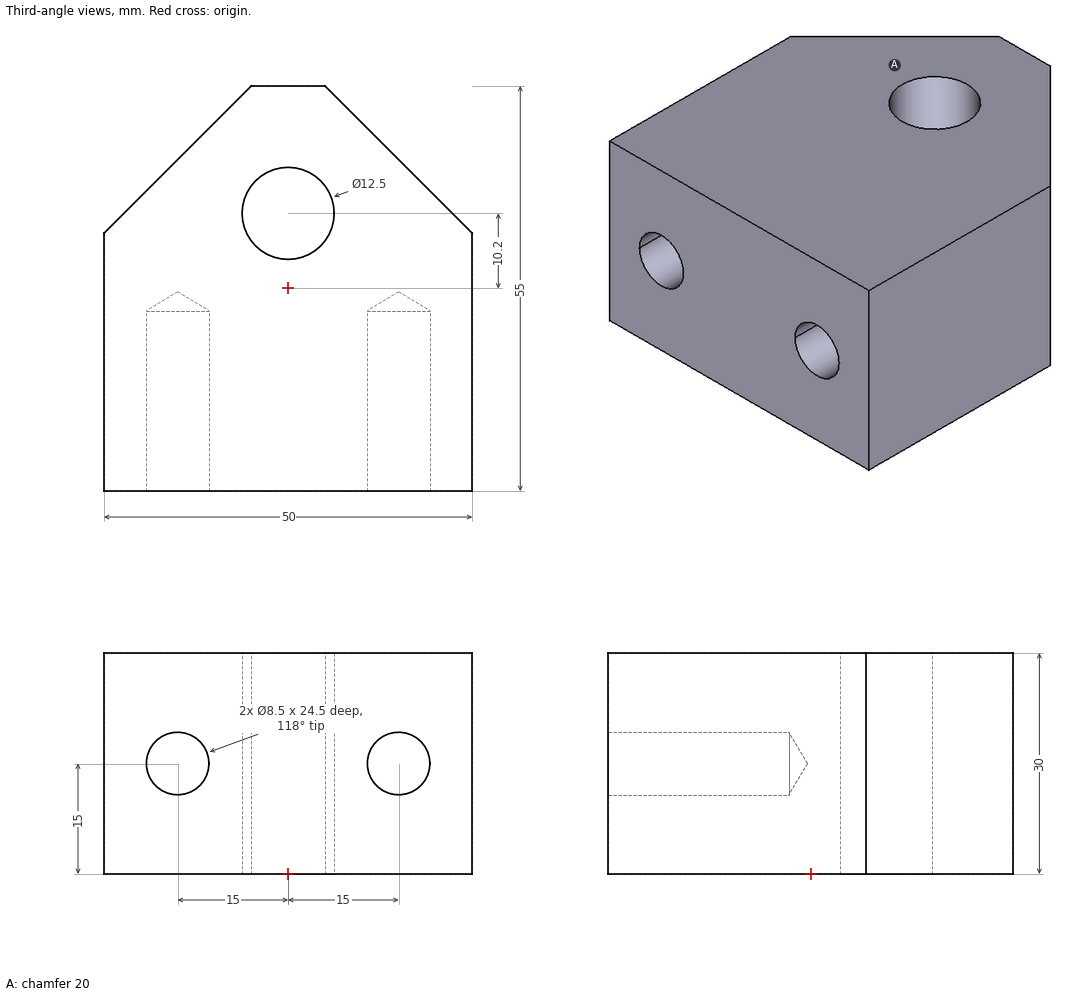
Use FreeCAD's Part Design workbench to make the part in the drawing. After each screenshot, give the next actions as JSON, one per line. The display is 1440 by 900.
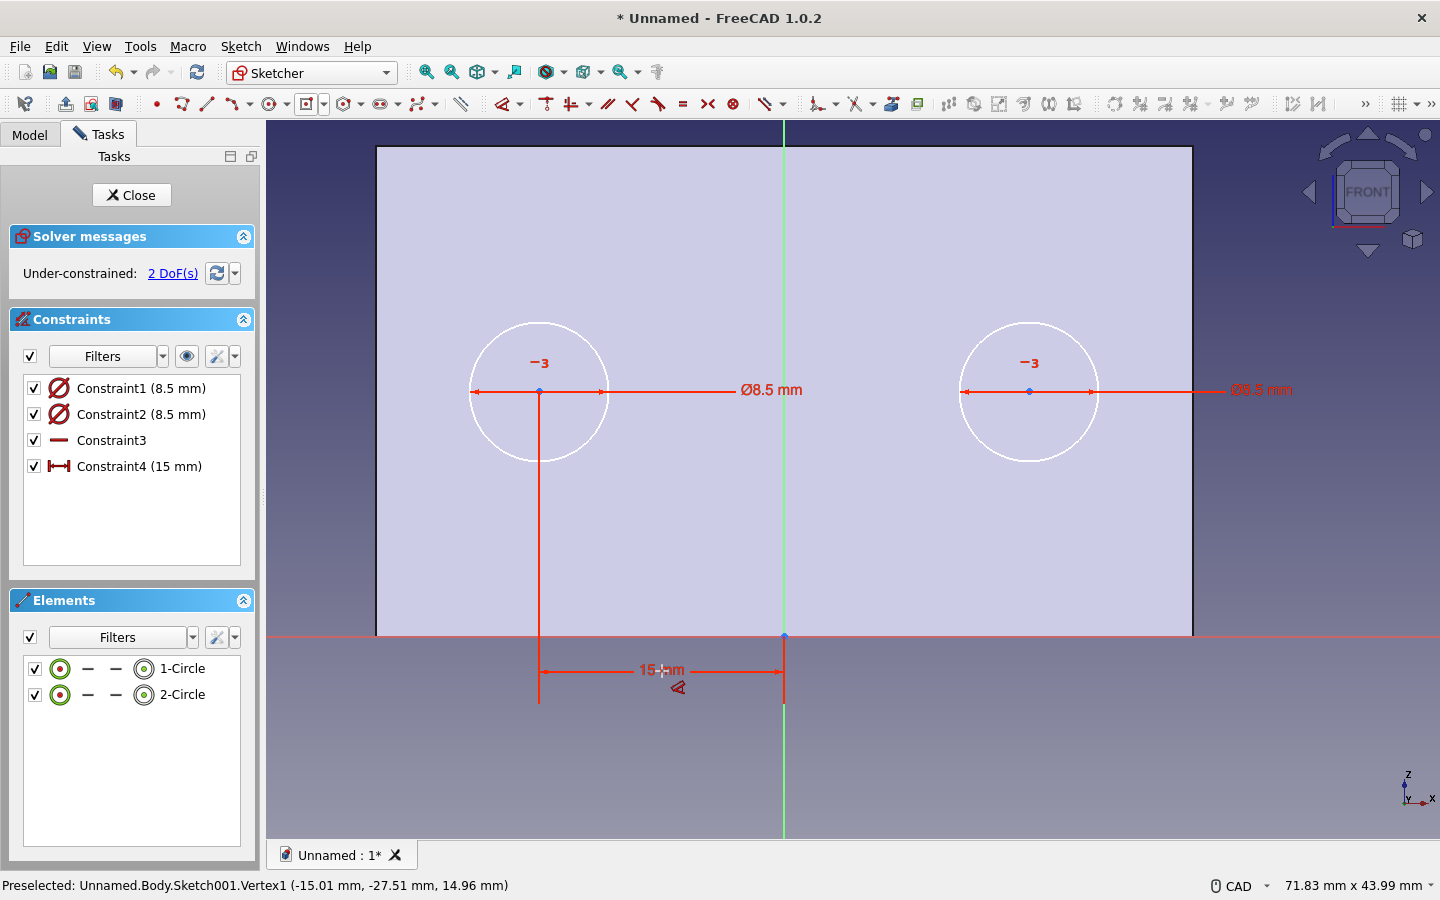
{"action": "left_click", "coordinate": [539, 392]}
{"action": "left_click", "coordinate": [505, 514]}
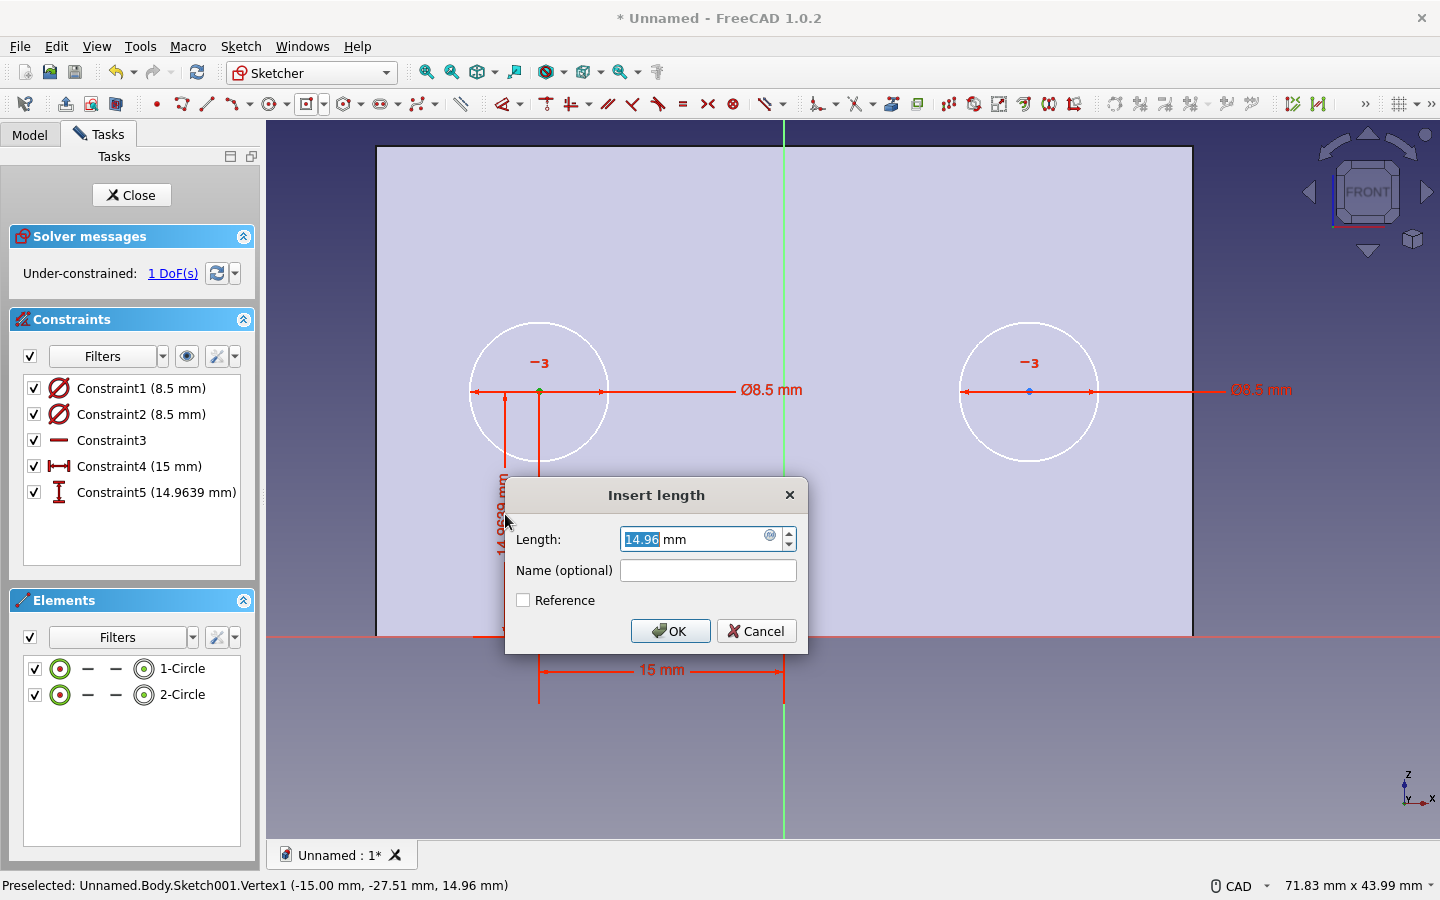
{"action": "type", "text": "15"}
{"action": "key", "text": "Return"}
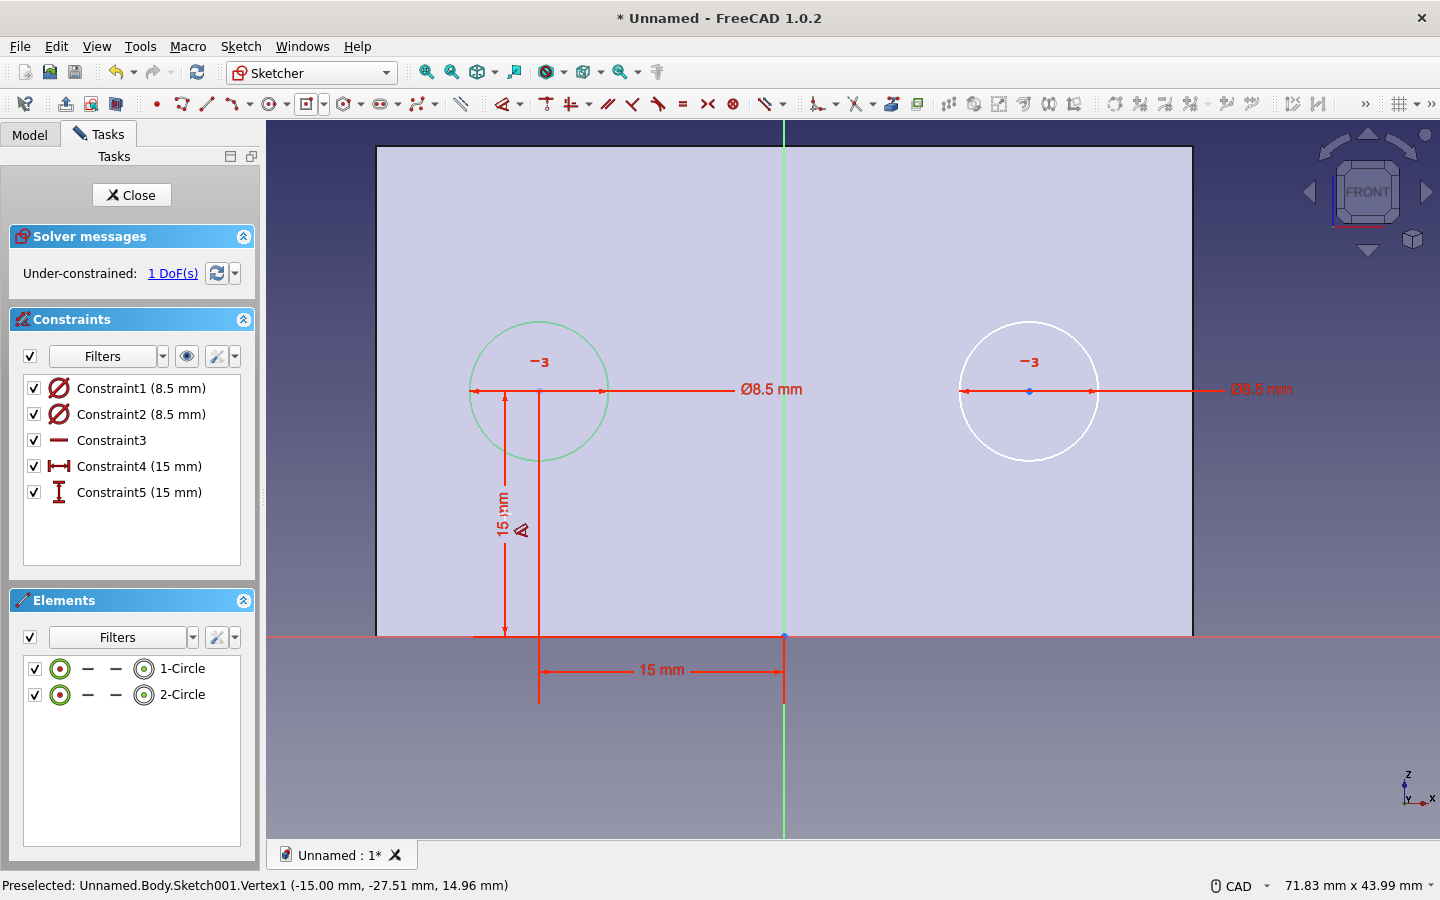
{"action": "left_click", "coordinate": [1029, 391]}
{"action": "left_click", "coordinate": [907, 671]}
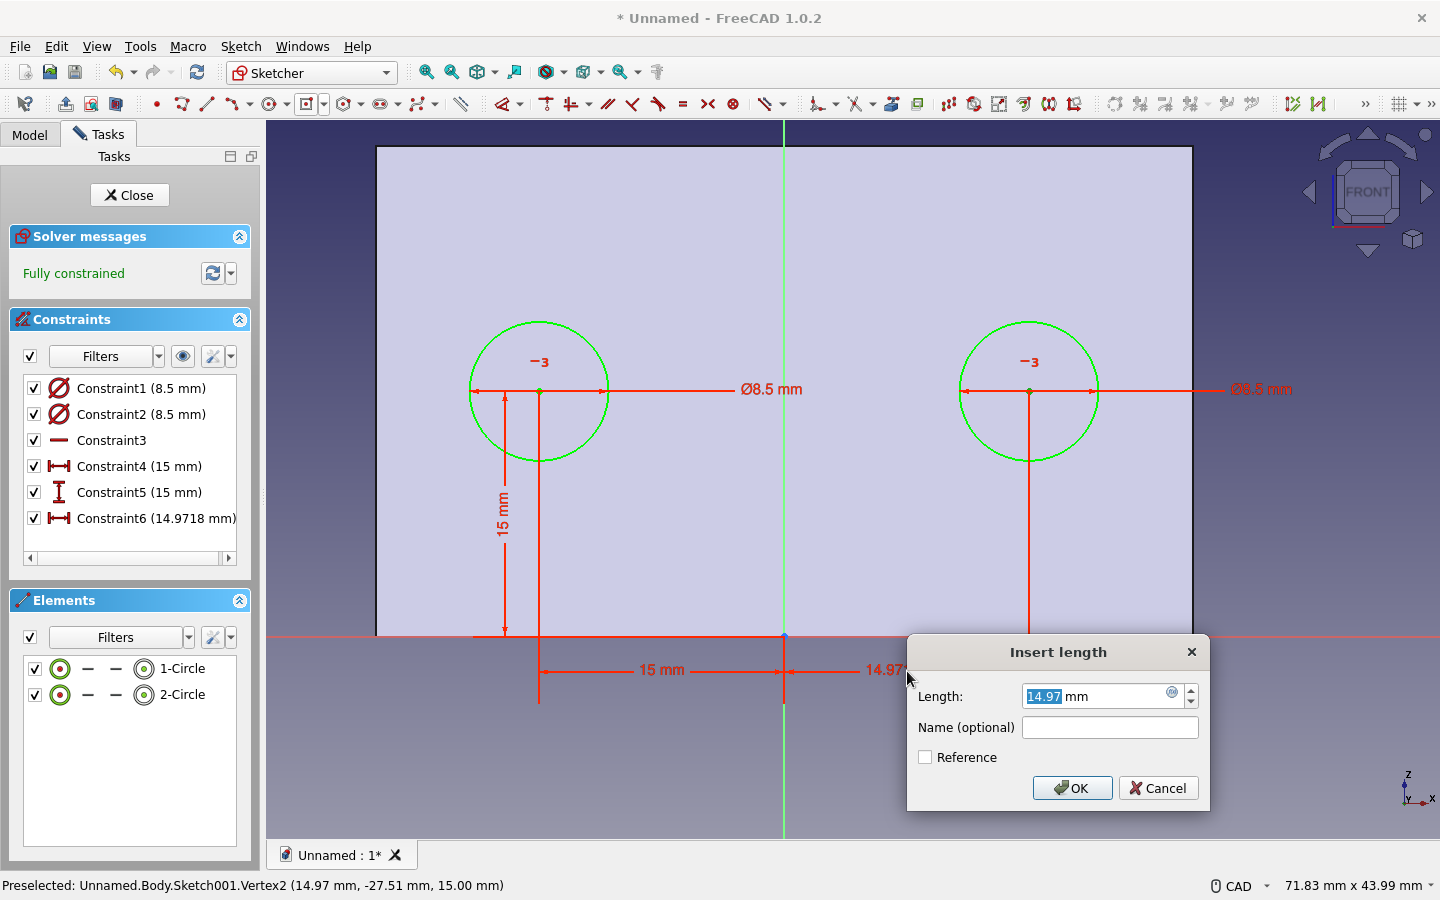
{"action": "type", "text": "15"}
{"action": "key", "text": "Return"}
{"action": "key", "text": "Escape"}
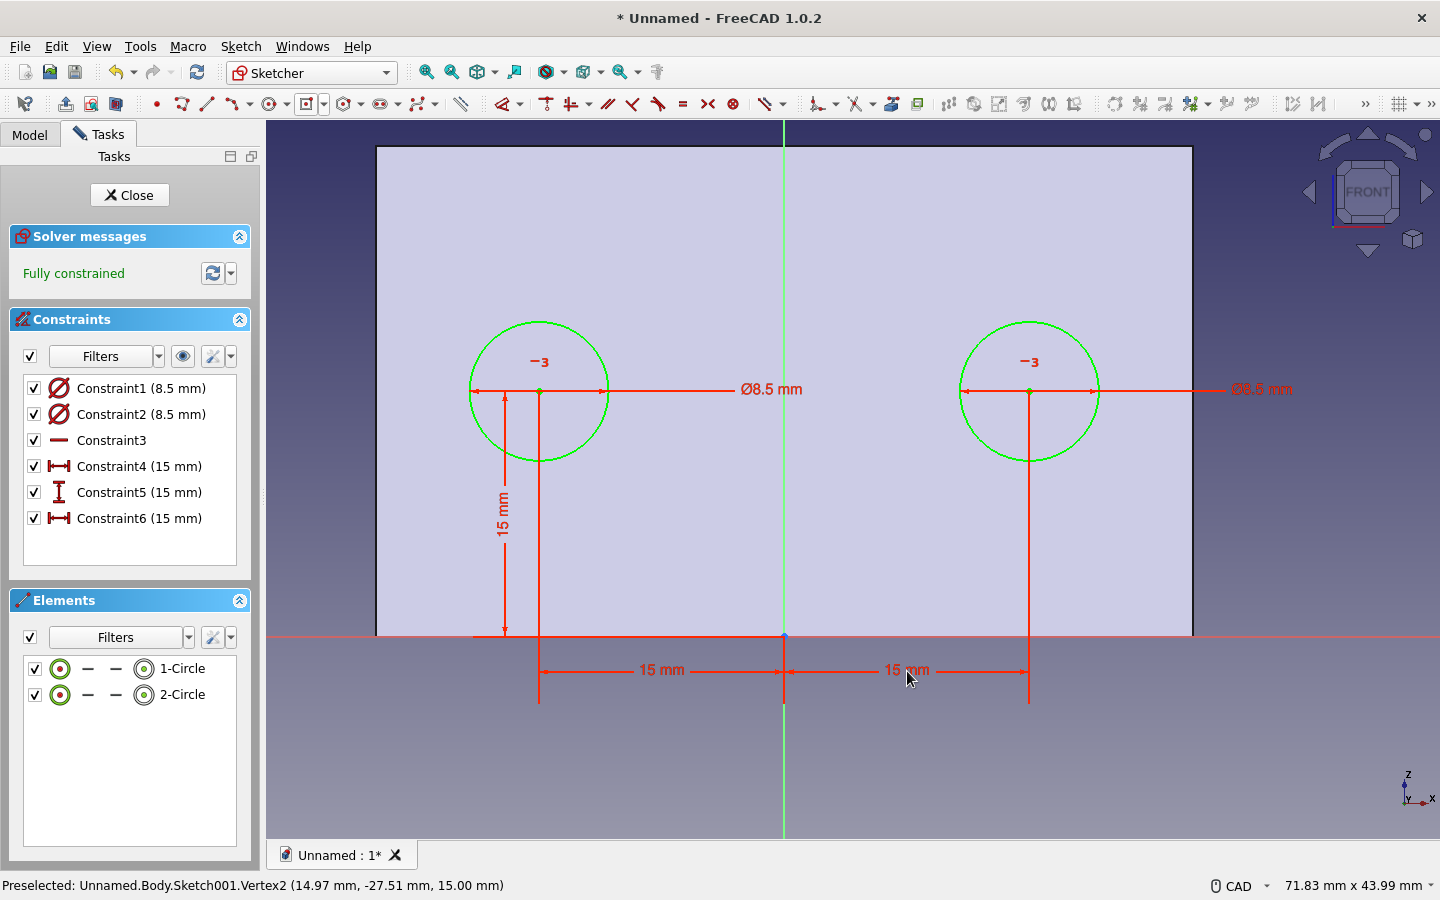
{"action": "left_click", "coordinate": [130, 195]}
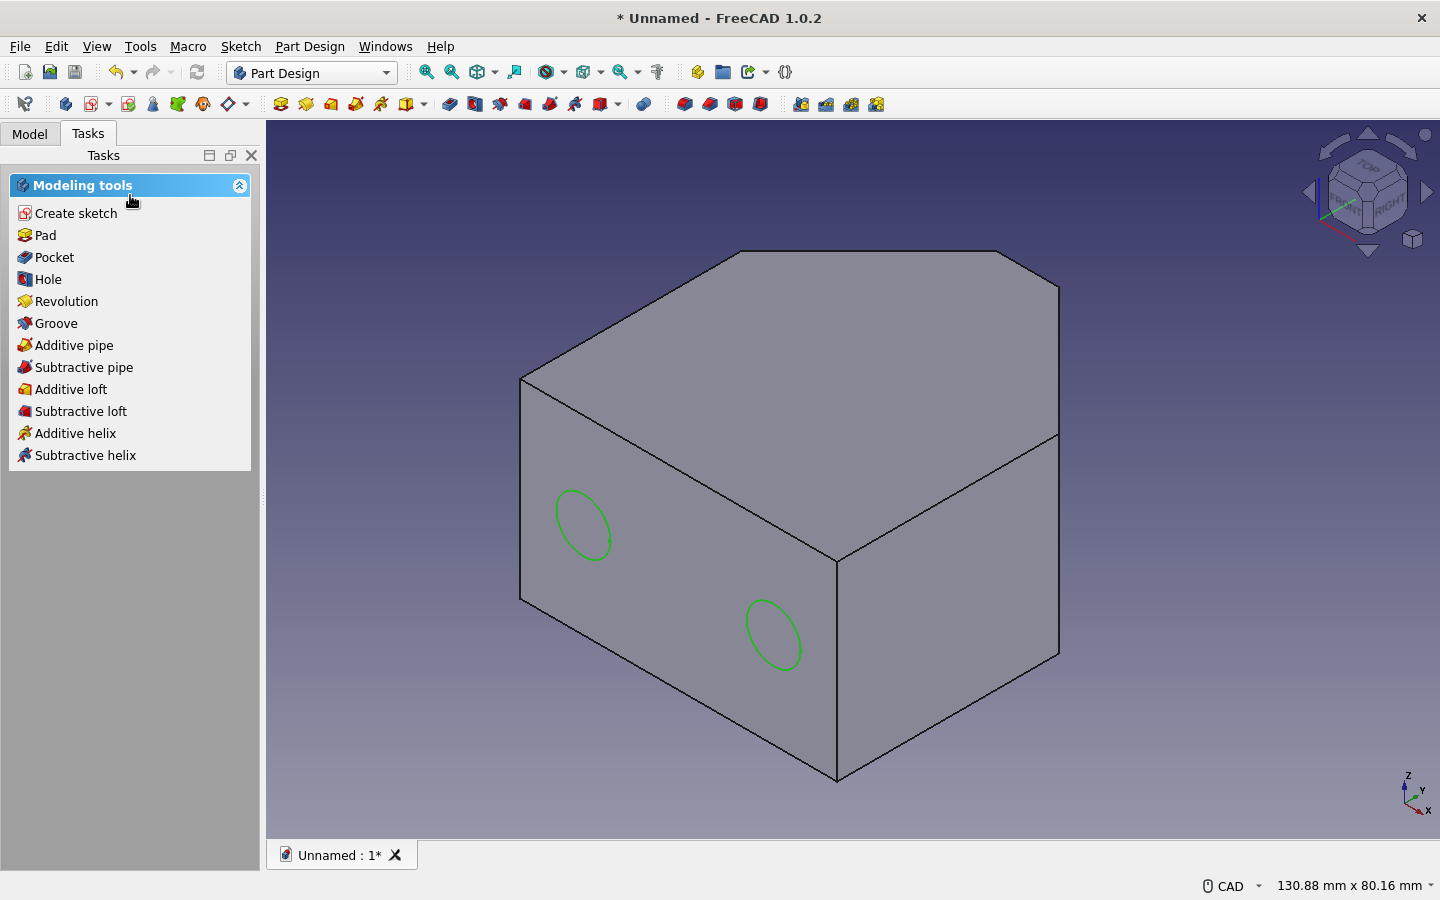
{"action": "left_click", "coordinate": [475, 104]}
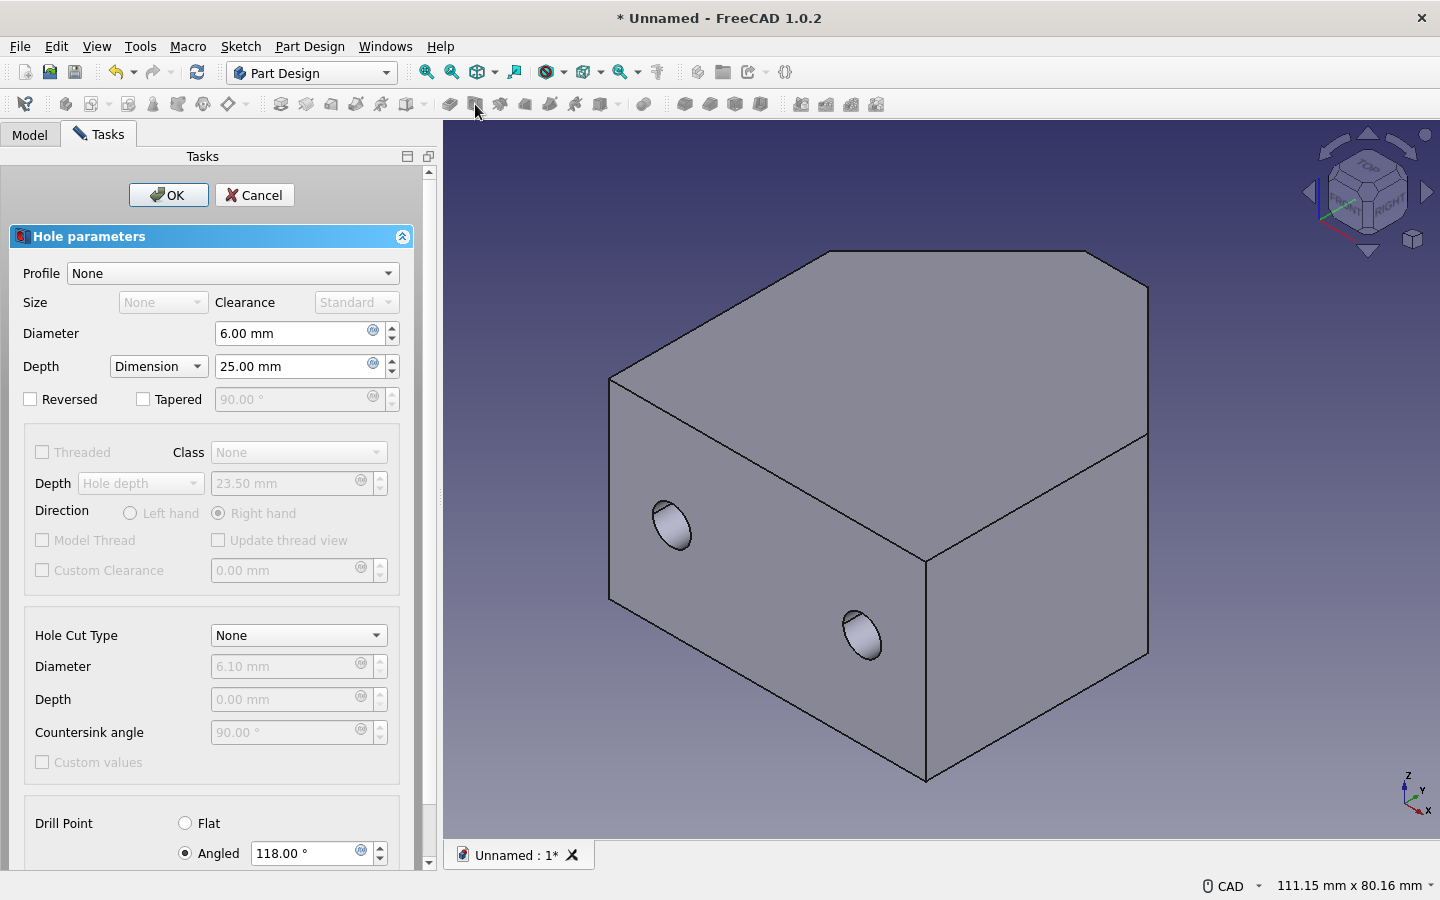
{"action": "triple_click", "coordinate": [300, 334]}